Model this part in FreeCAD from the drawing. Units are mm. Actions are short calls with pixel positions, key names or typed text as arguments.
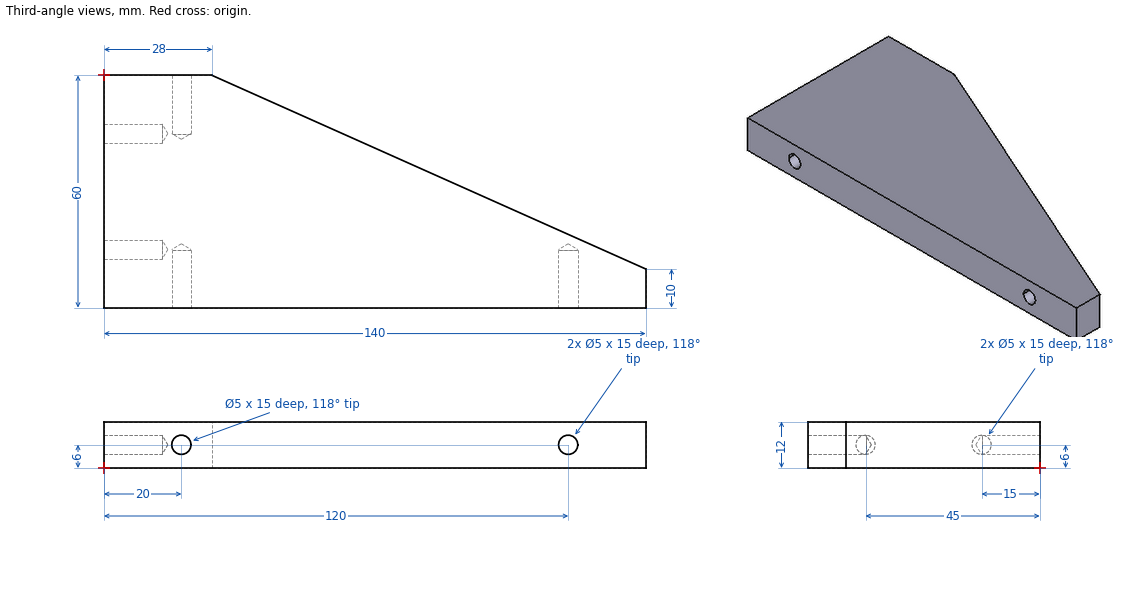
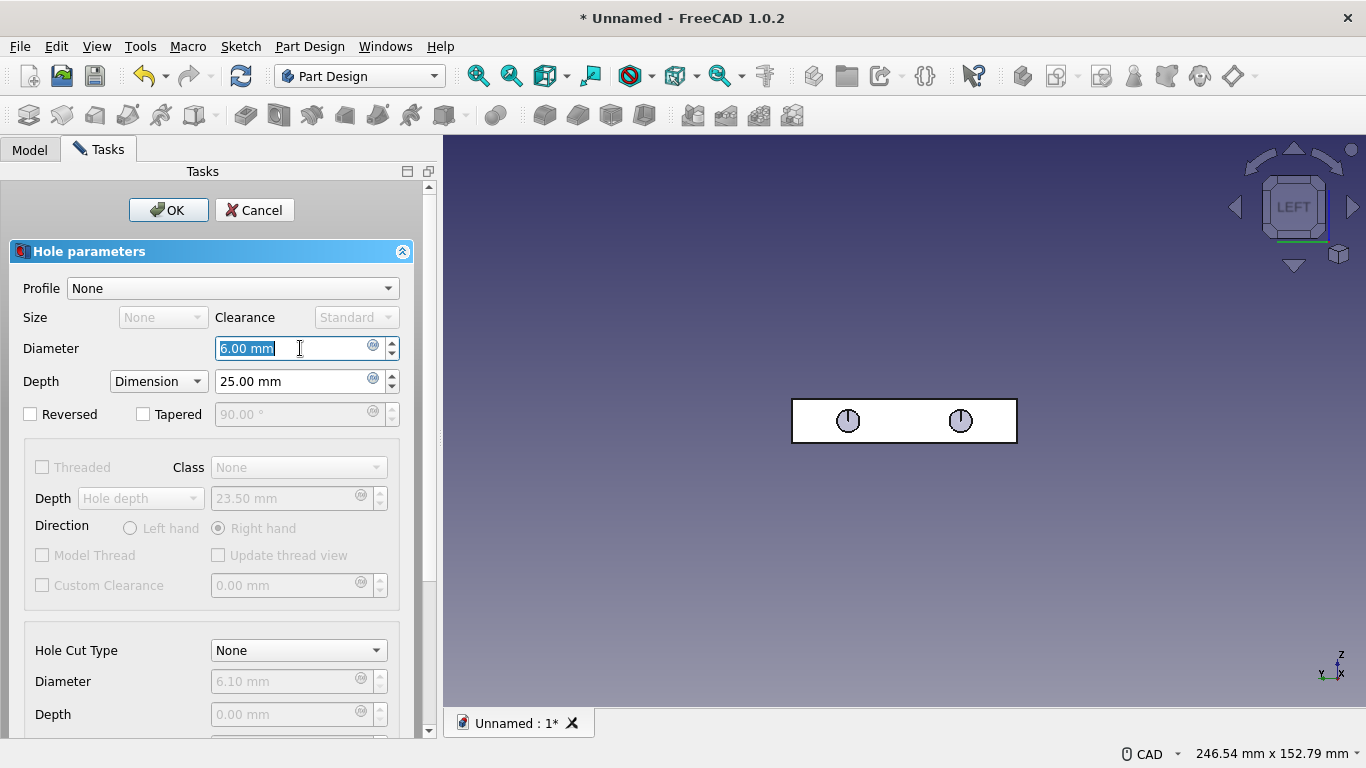
text(5)
key(Tab)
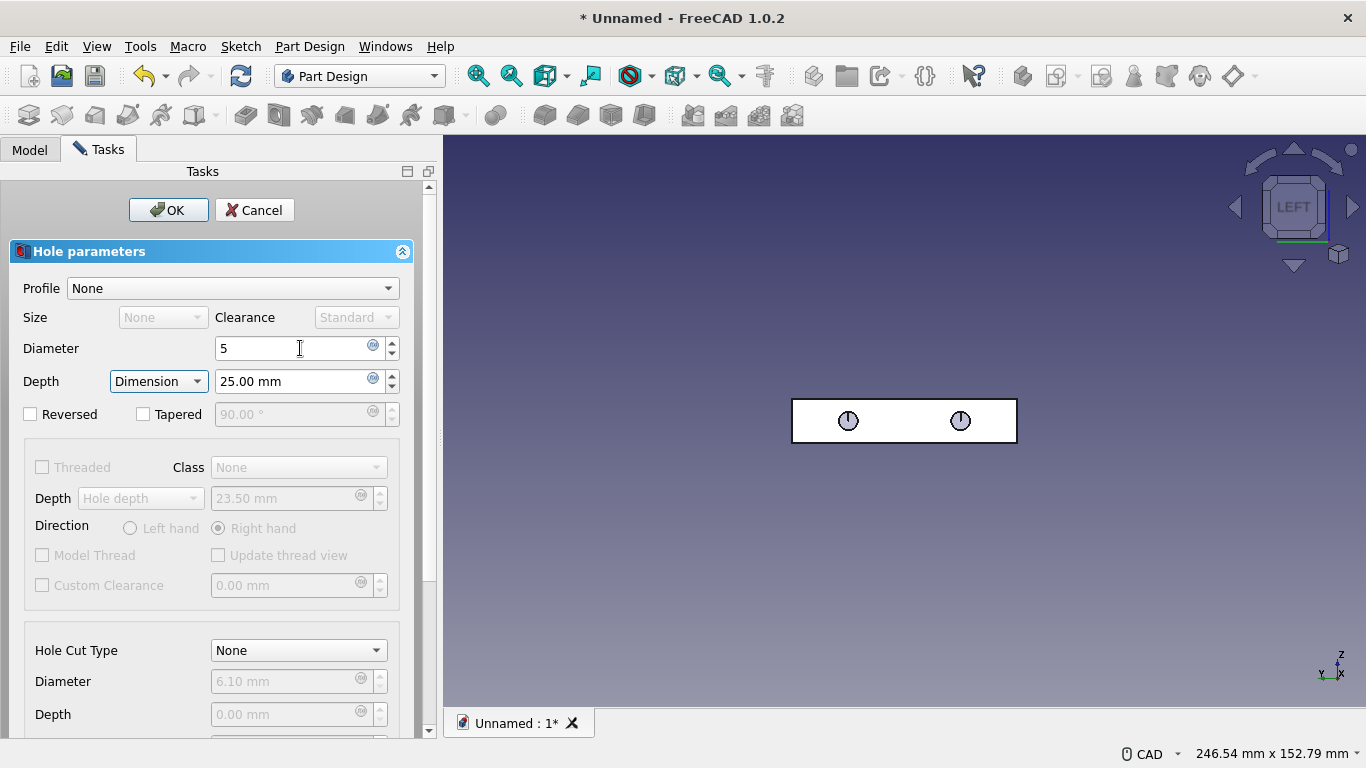
triple_click(300, 382)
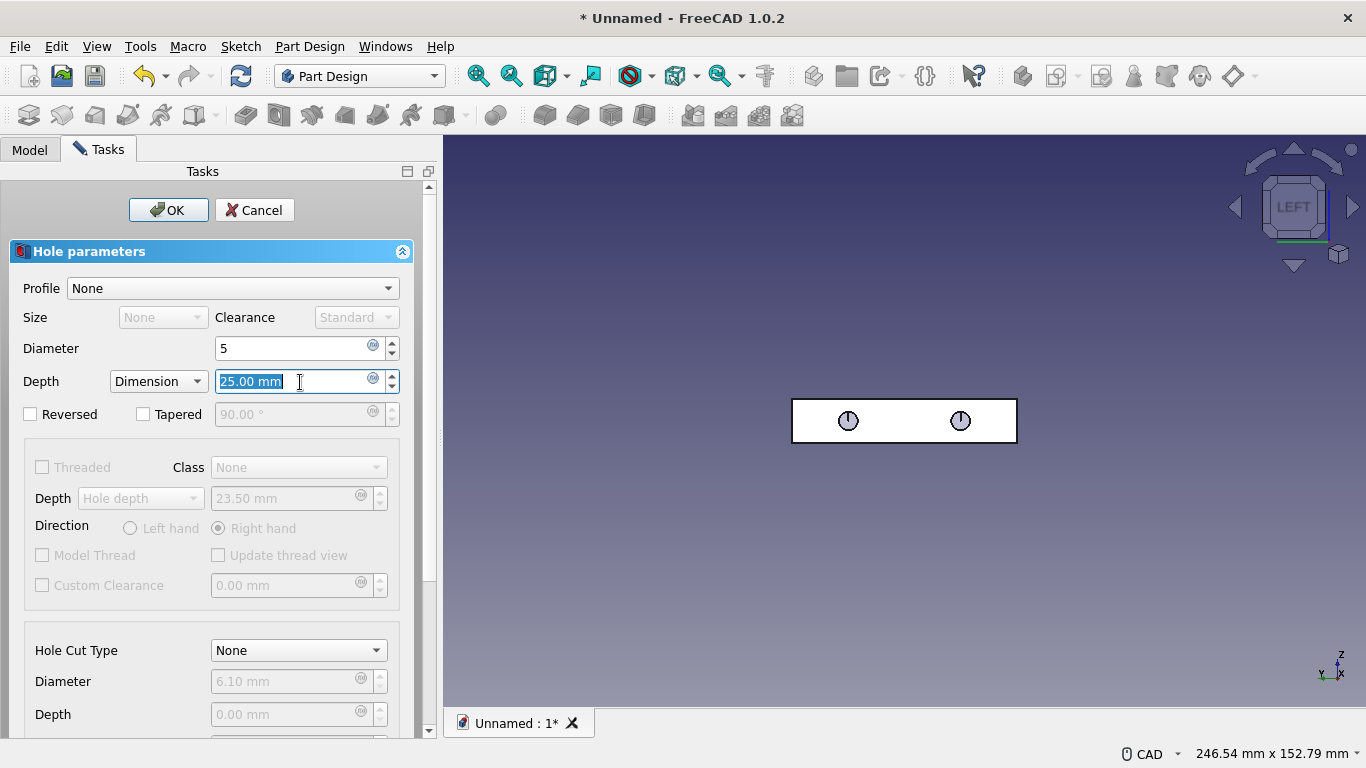
text(15)
key(Tab)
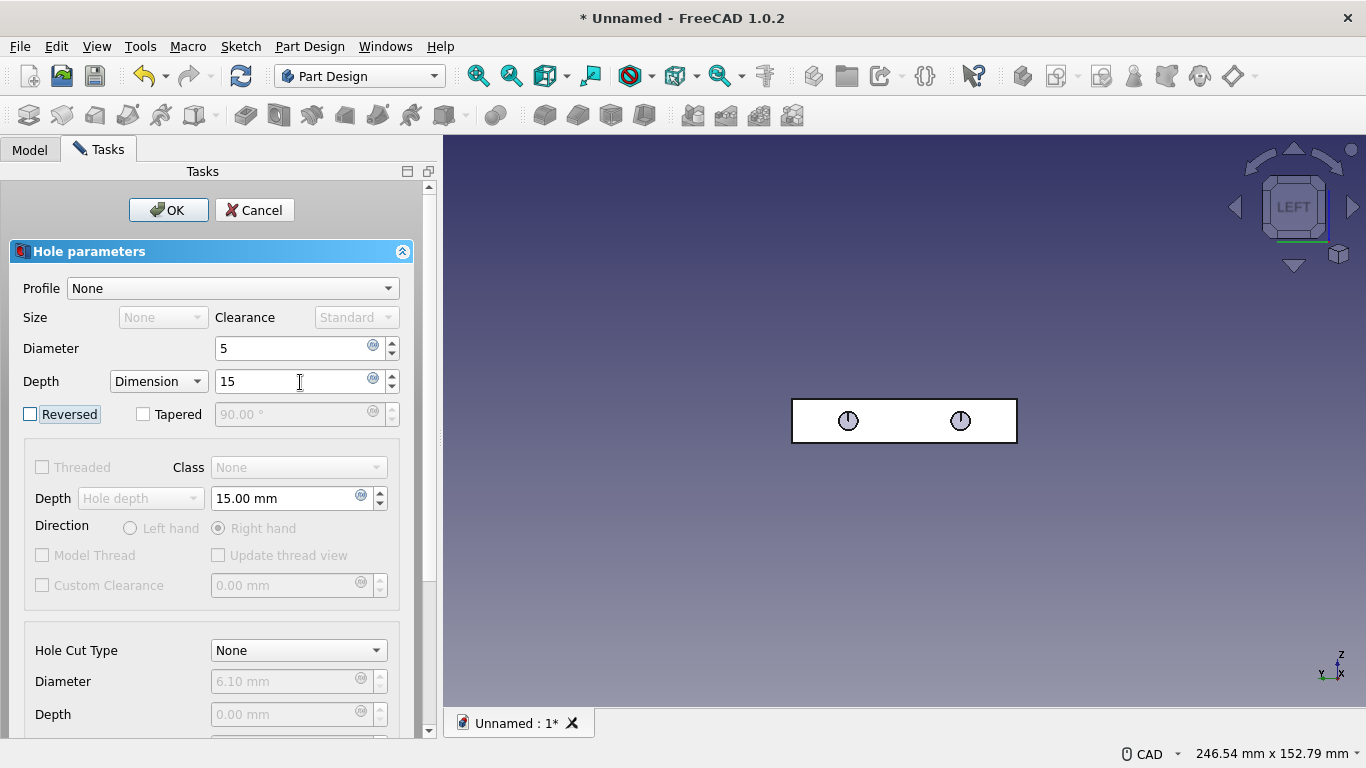
click(169, 210)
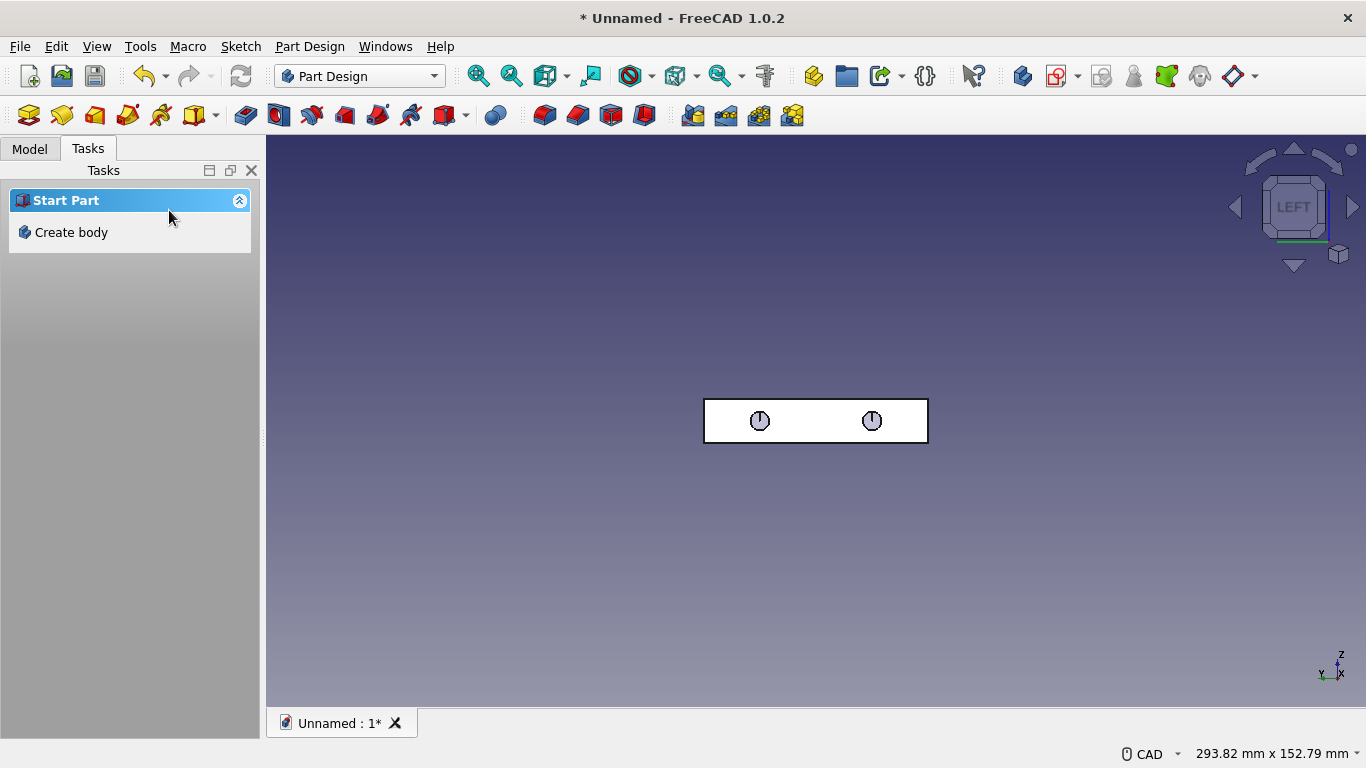
key(v)
key(f)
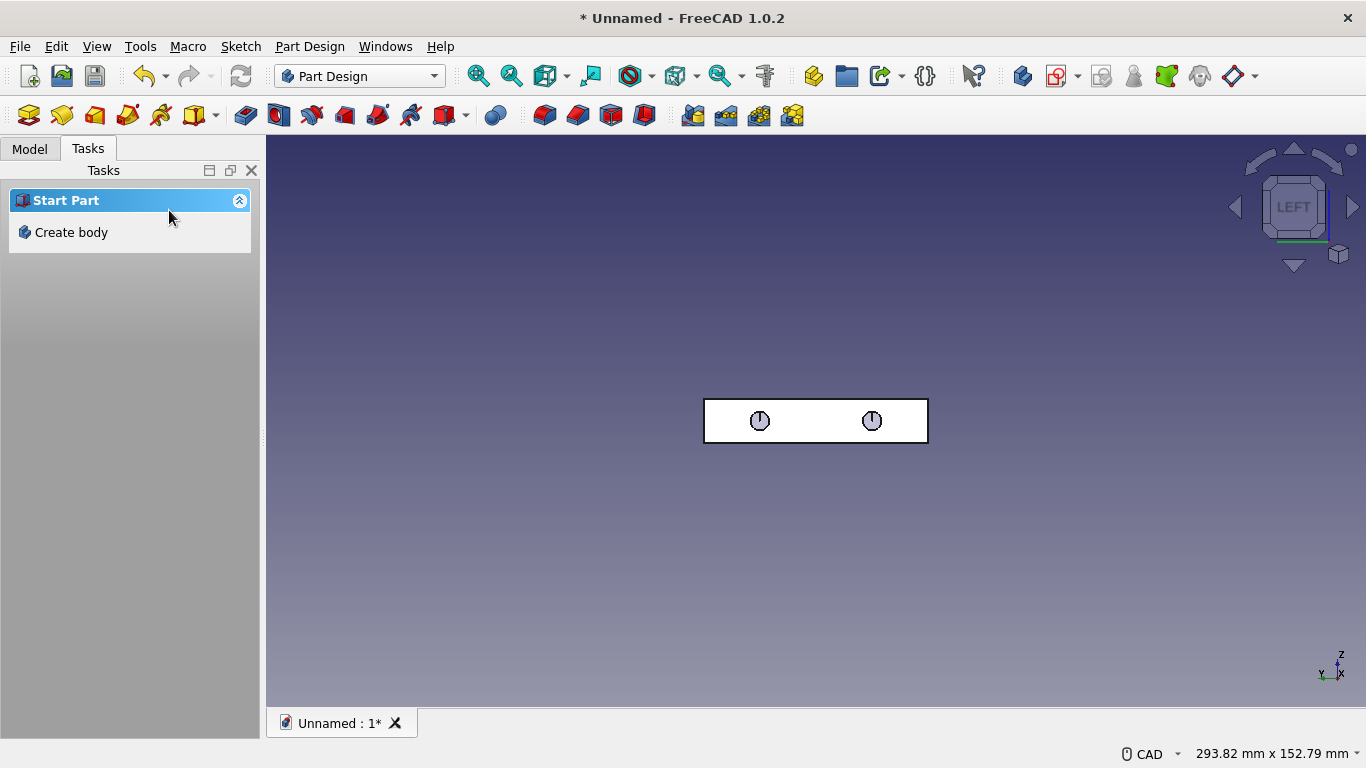
key(0)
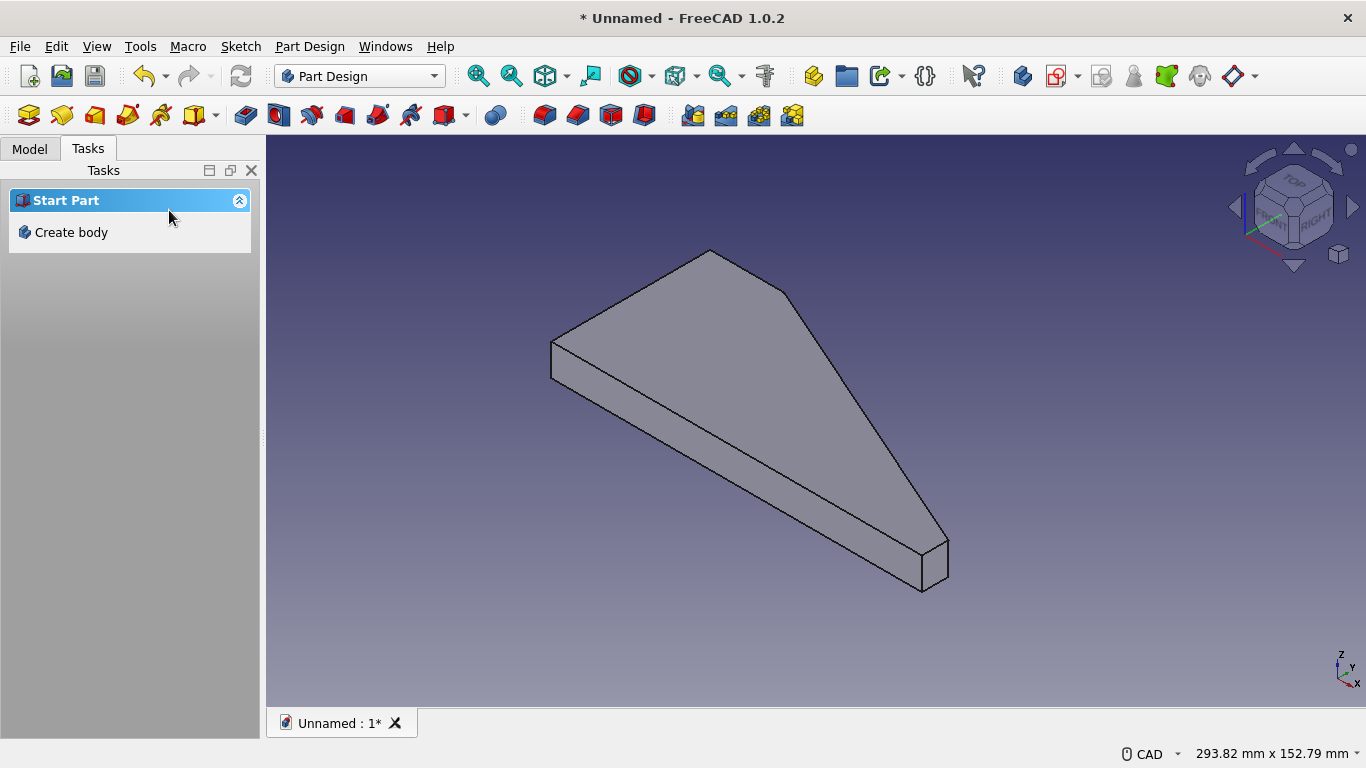
click(895, 558)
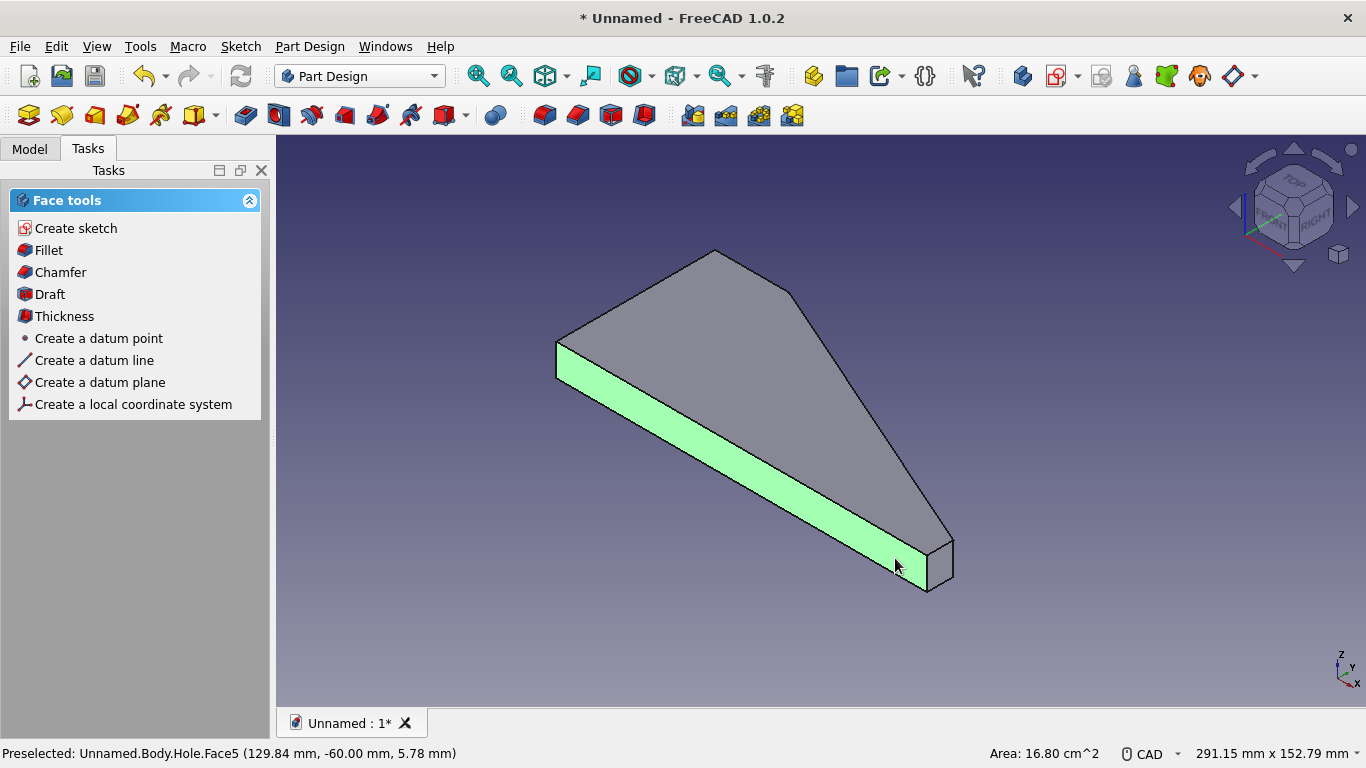
click(1056, 76)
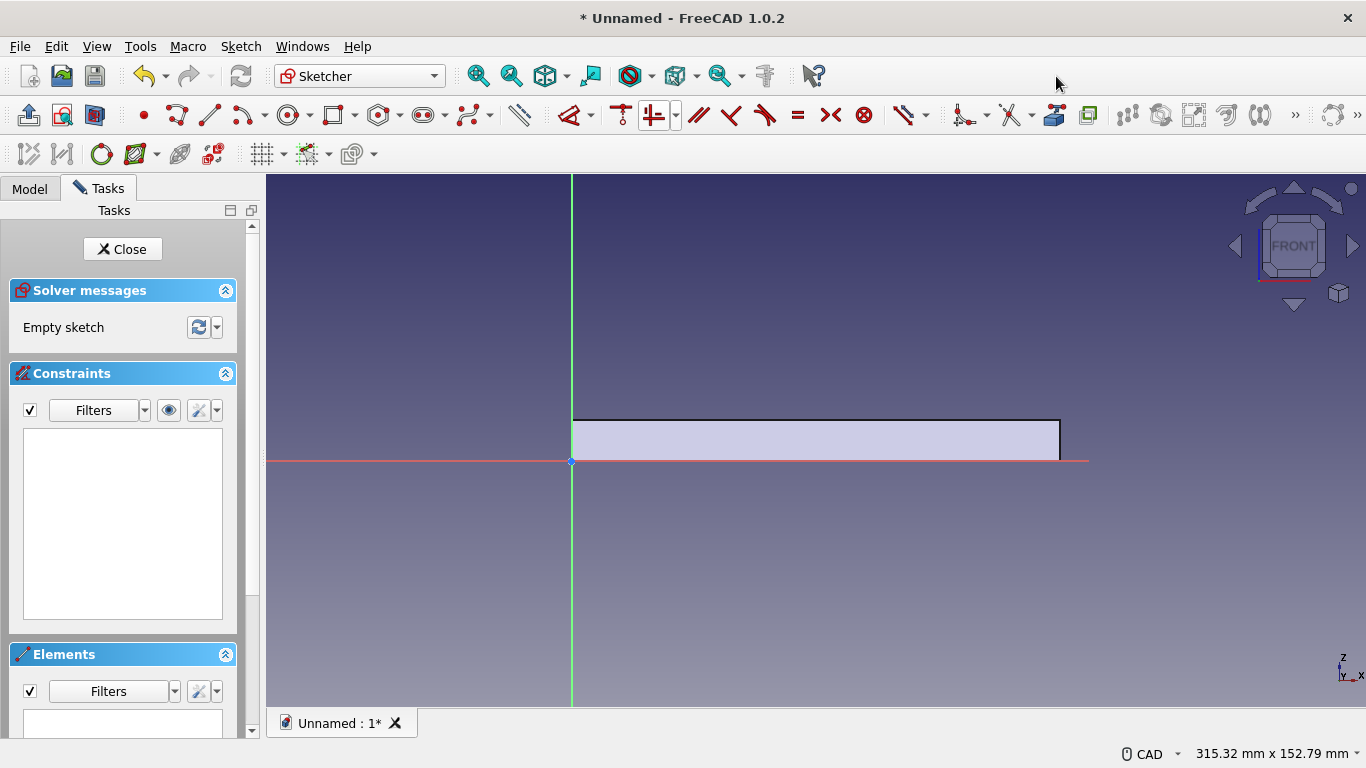
scroll(863, 459, up, 2)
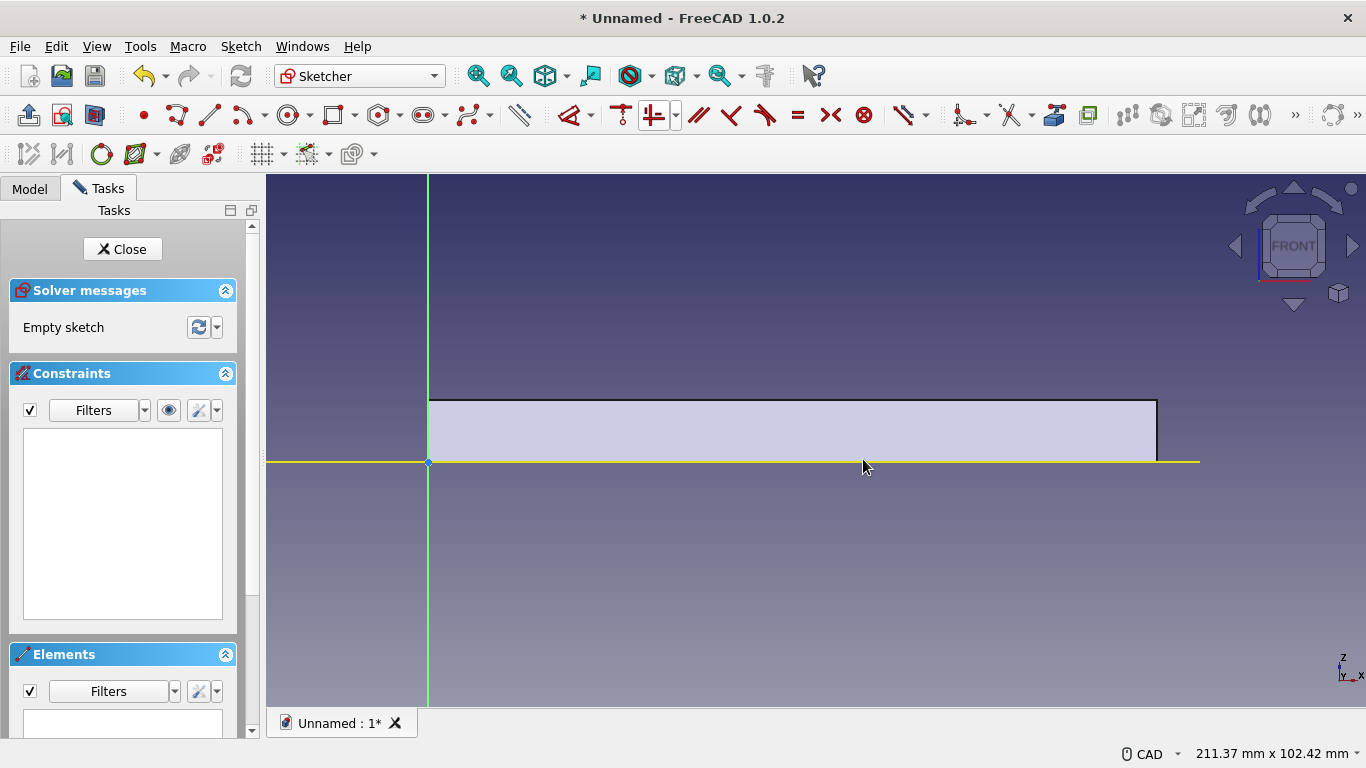
key(g)
key(c)